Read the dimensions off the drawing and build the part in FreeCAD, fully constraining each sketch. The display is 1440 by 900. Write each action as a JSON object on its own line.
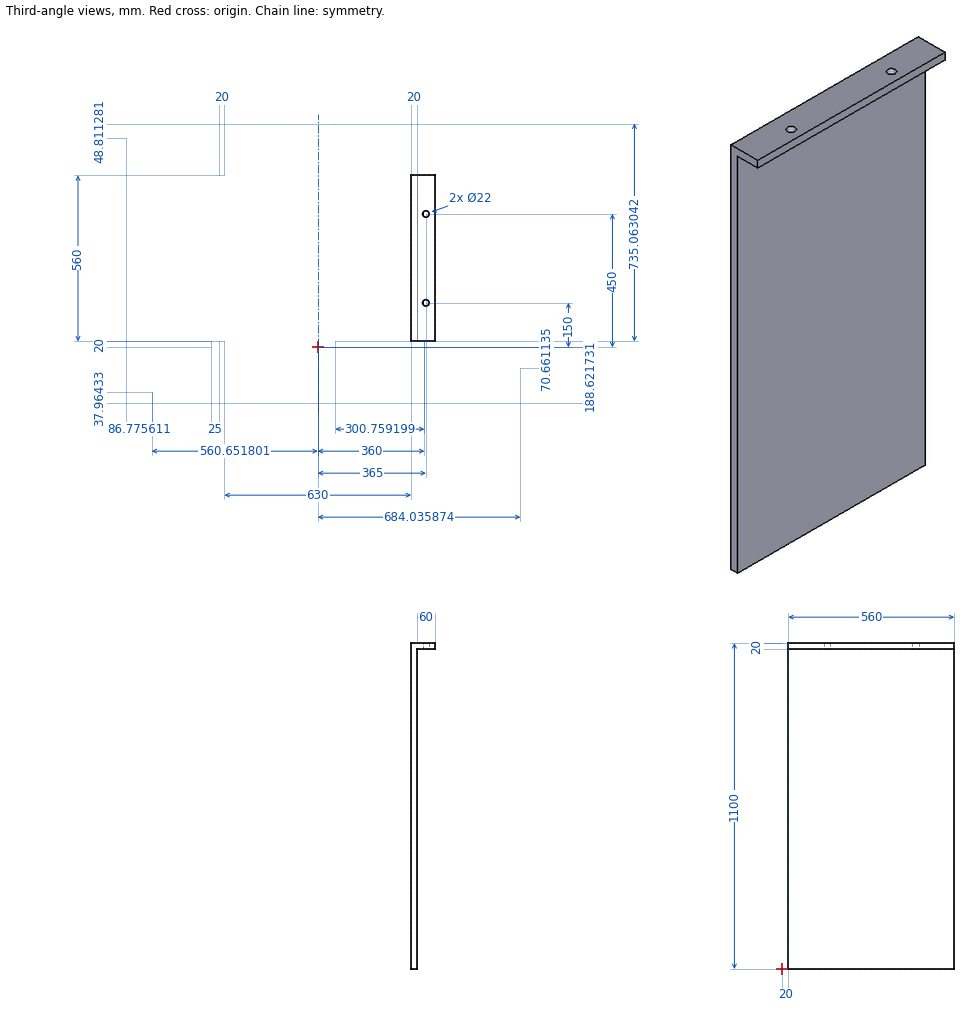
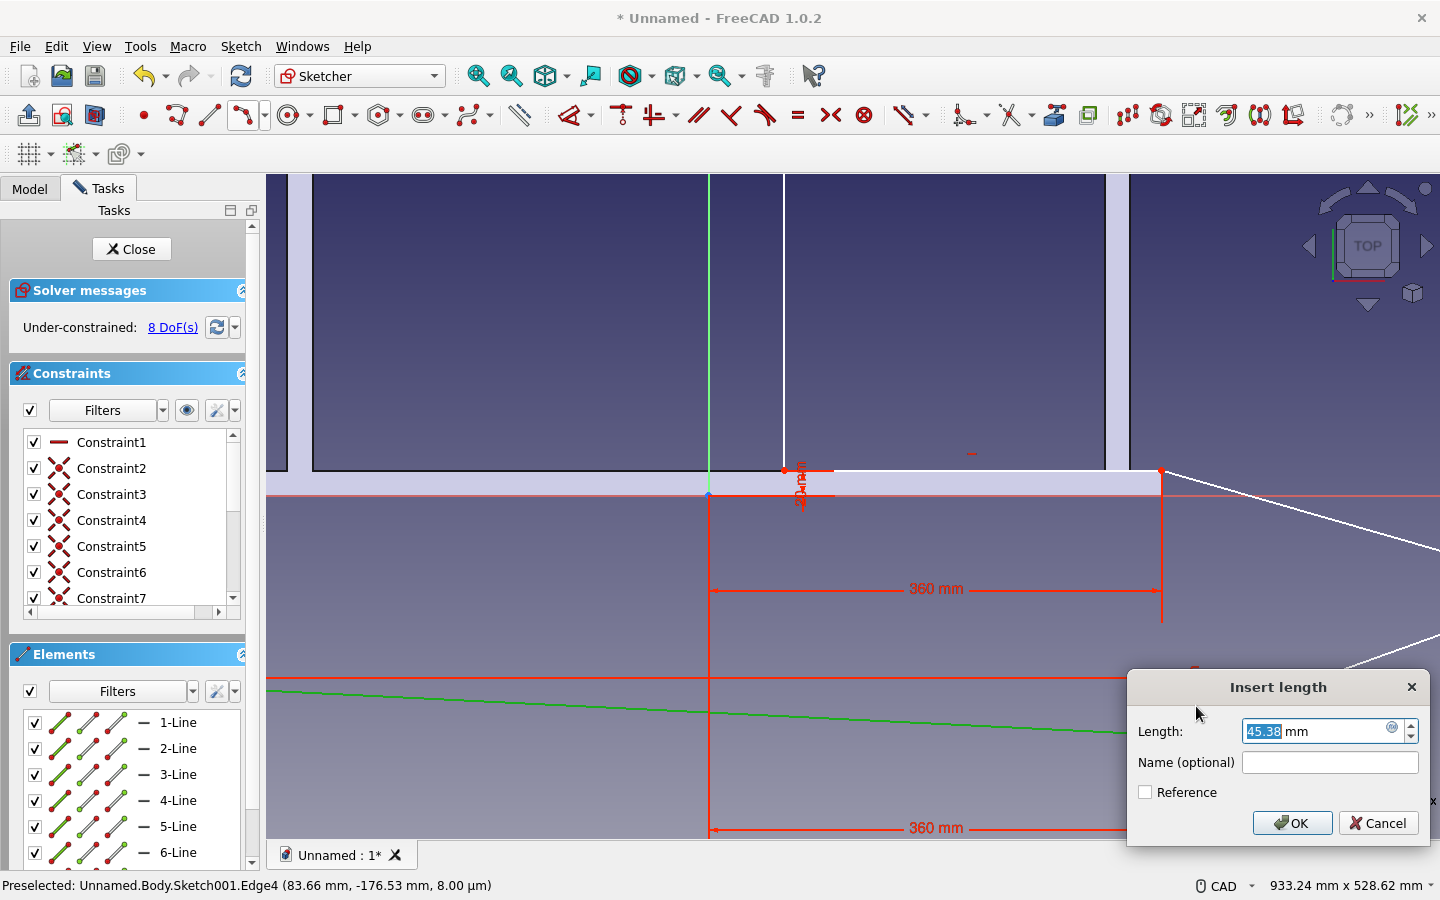
{"action": "type", "text": "37.96433"}
{"action": "key", "text": "Return"}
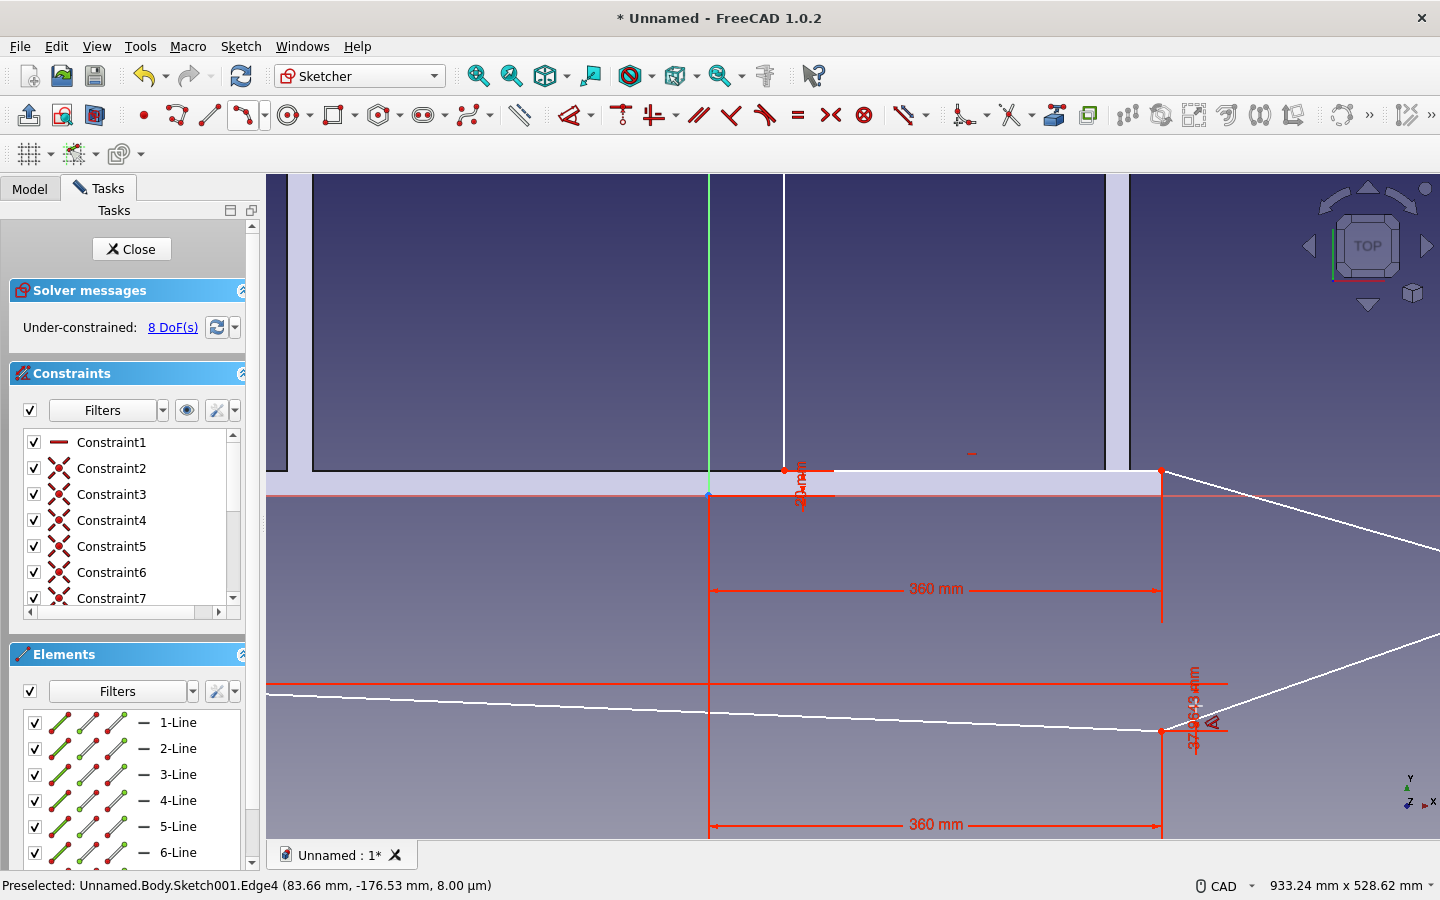
{"action": "left_click", "coordinate": [898, 471]}
{"action": "left_click", "coordinate": [973, 437]}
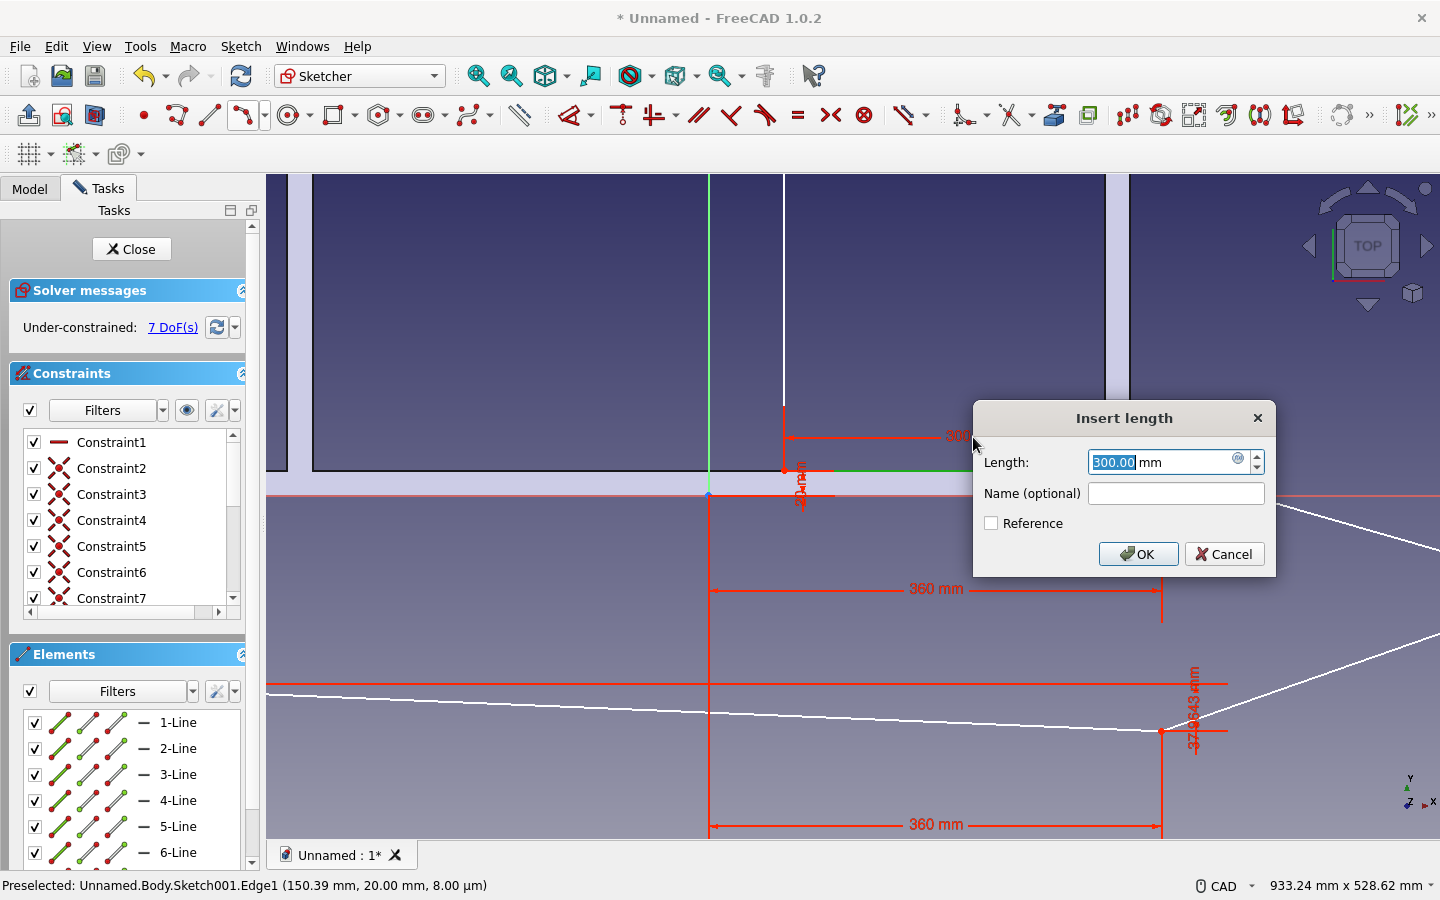
{"action": "type", "text": "300.759199"}
{"action": "key", "text": "Return"}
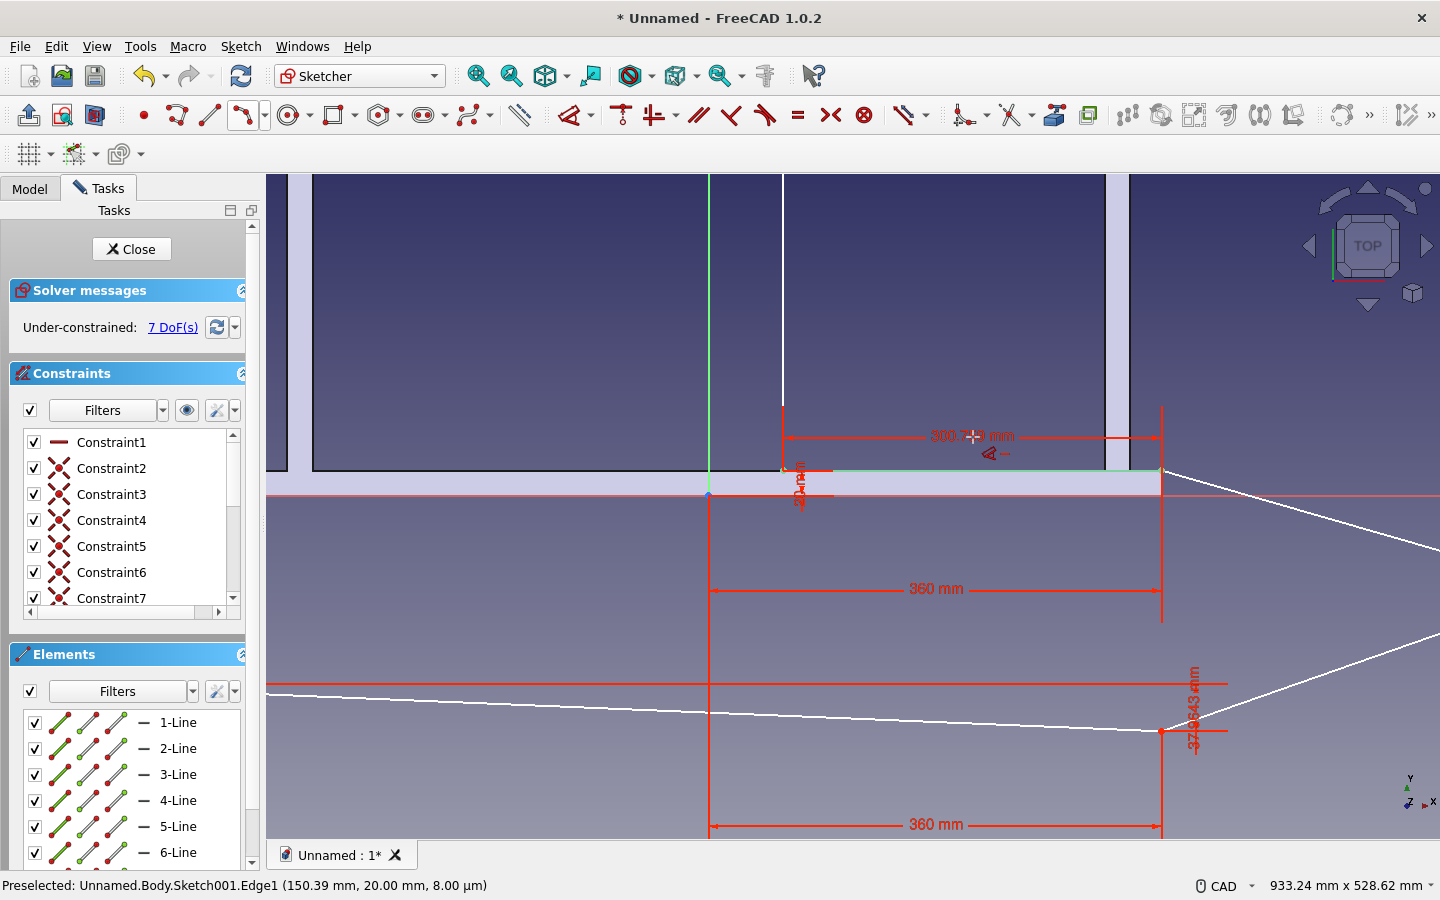
{"action": "left_click", "coordinate": [783, 286]}
{"action": "left_click", "coordinate": [817, 336]}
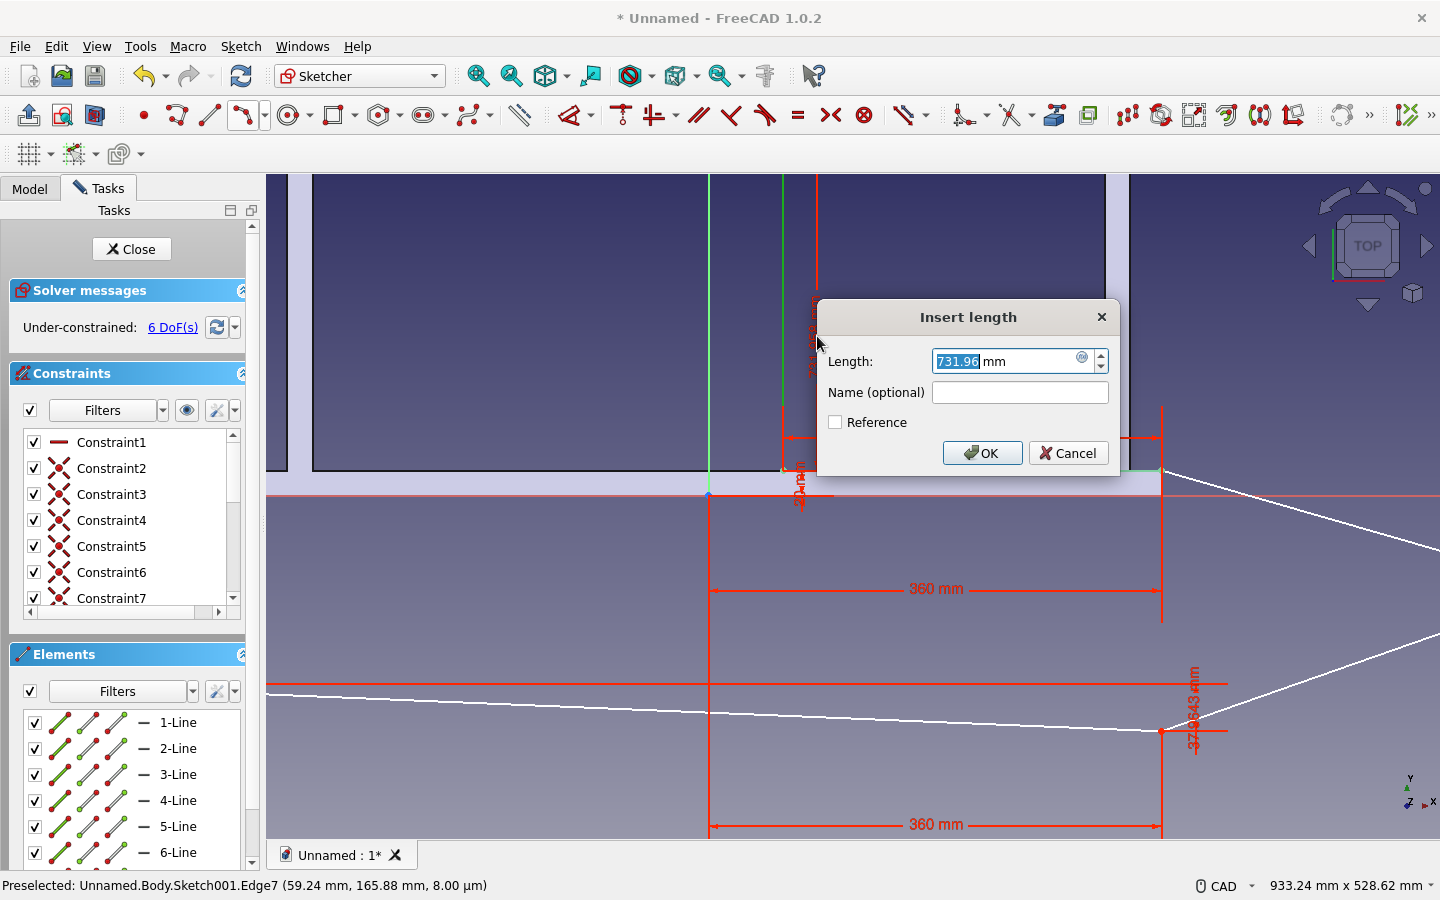
{"action": "type", "text": "735.063042"}
{"action": "key", "text": "Return"}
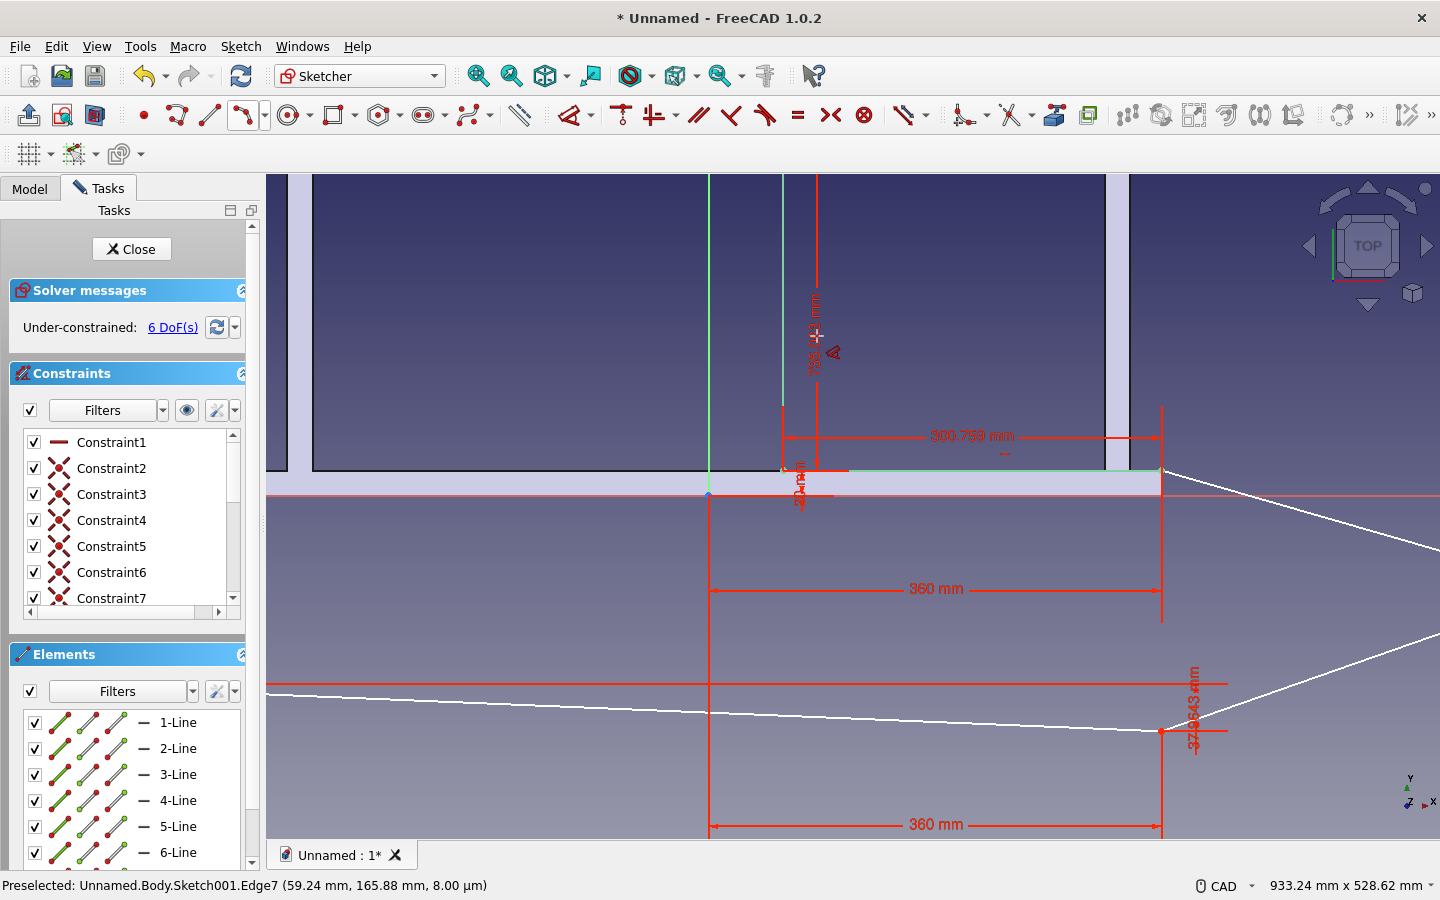
{"action": "scroll", "coordinate": [815, 720], "scroll_direction": "down", "scroll_amount": 5}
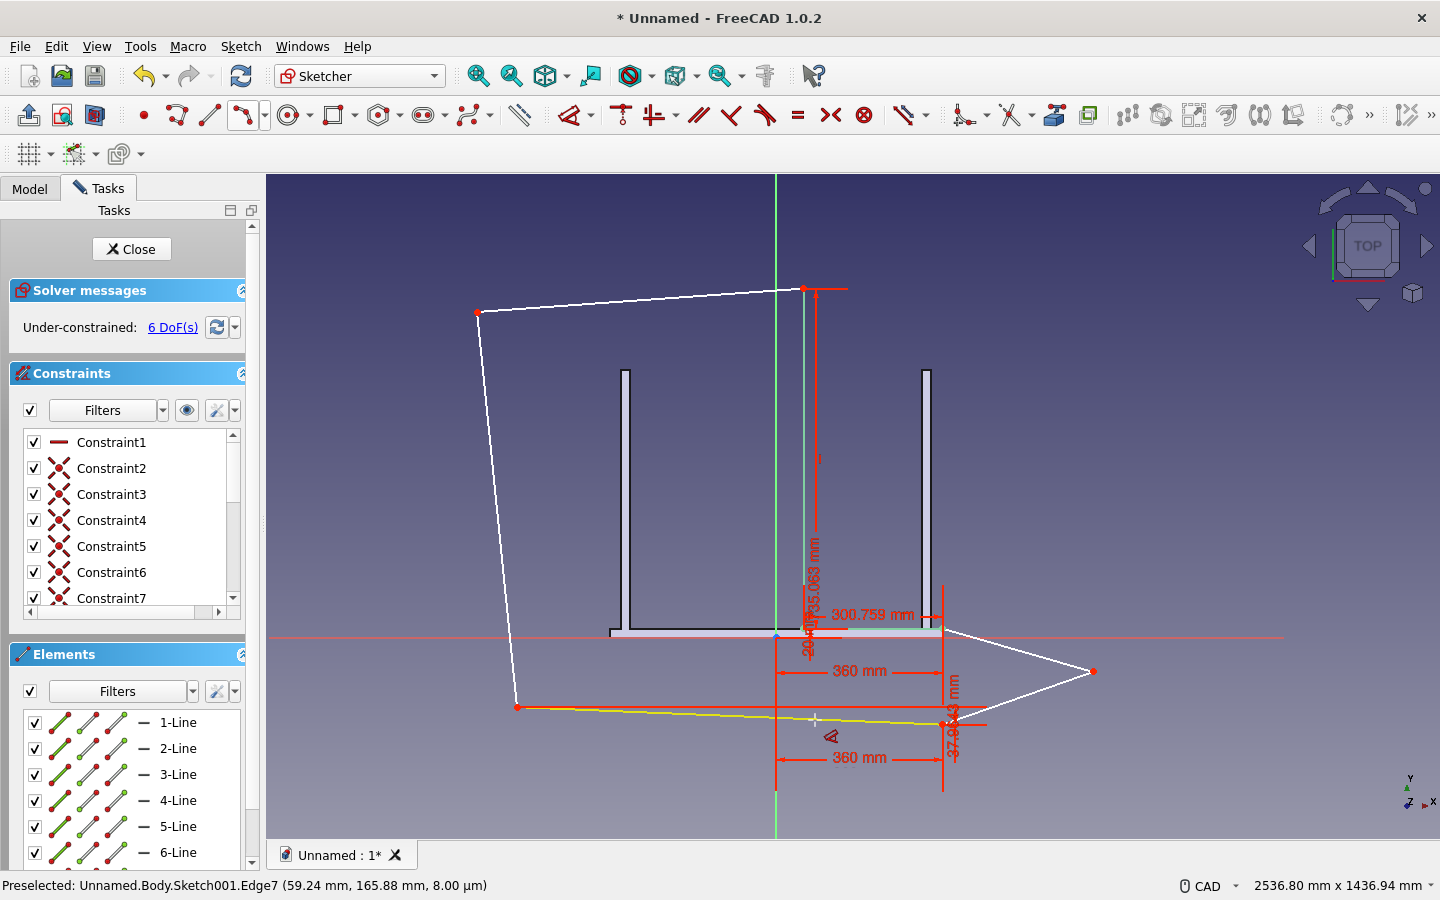
{"action": "left_click", "coordinate": [1093, 672]}
{"action": "left_click", "coordinate": [1127, 655]}